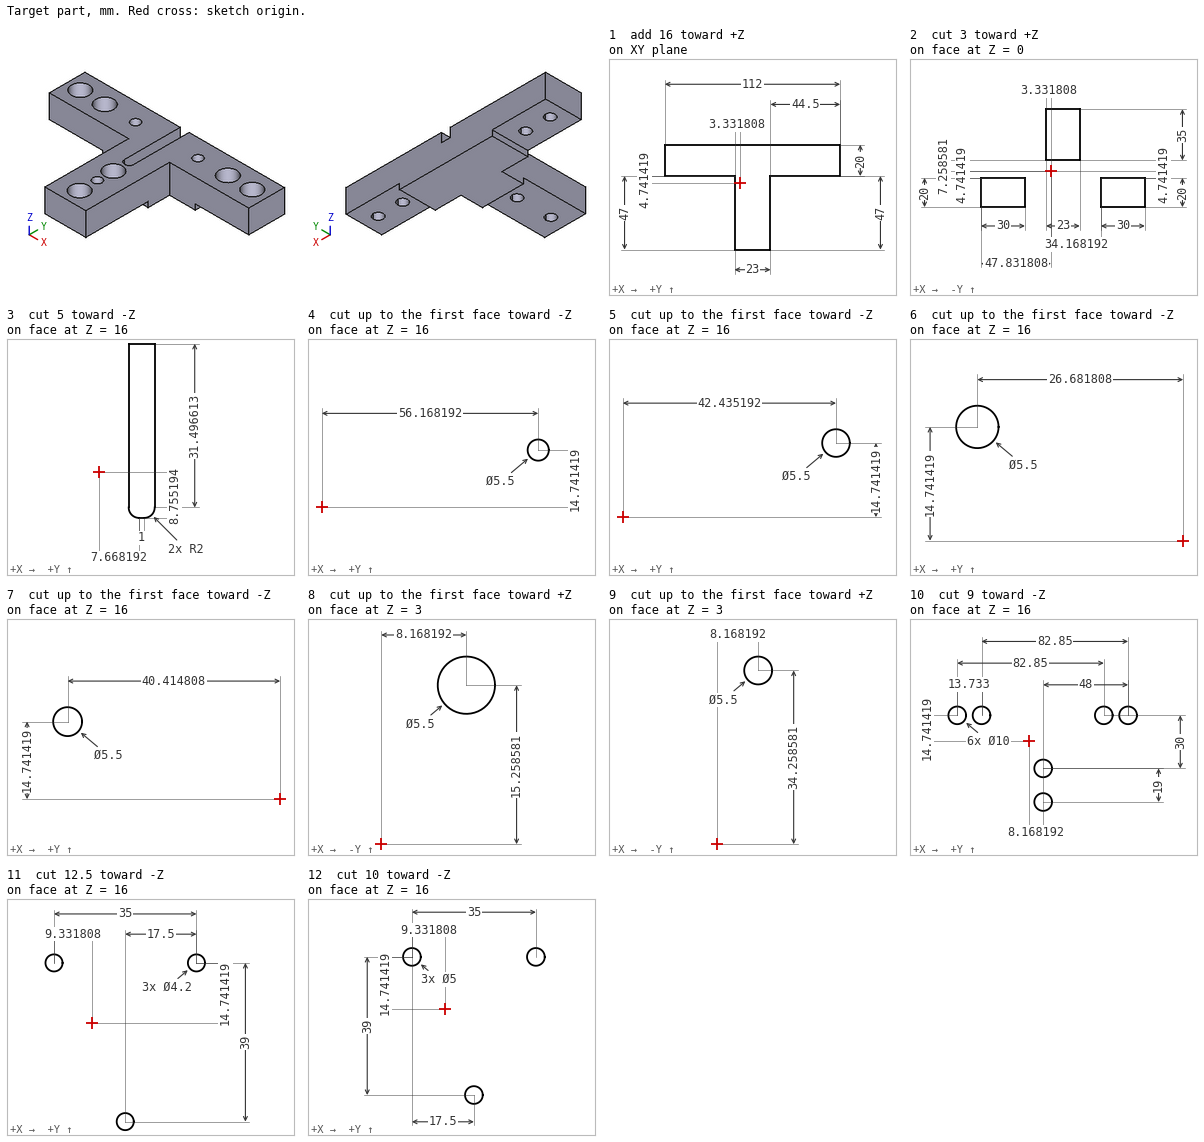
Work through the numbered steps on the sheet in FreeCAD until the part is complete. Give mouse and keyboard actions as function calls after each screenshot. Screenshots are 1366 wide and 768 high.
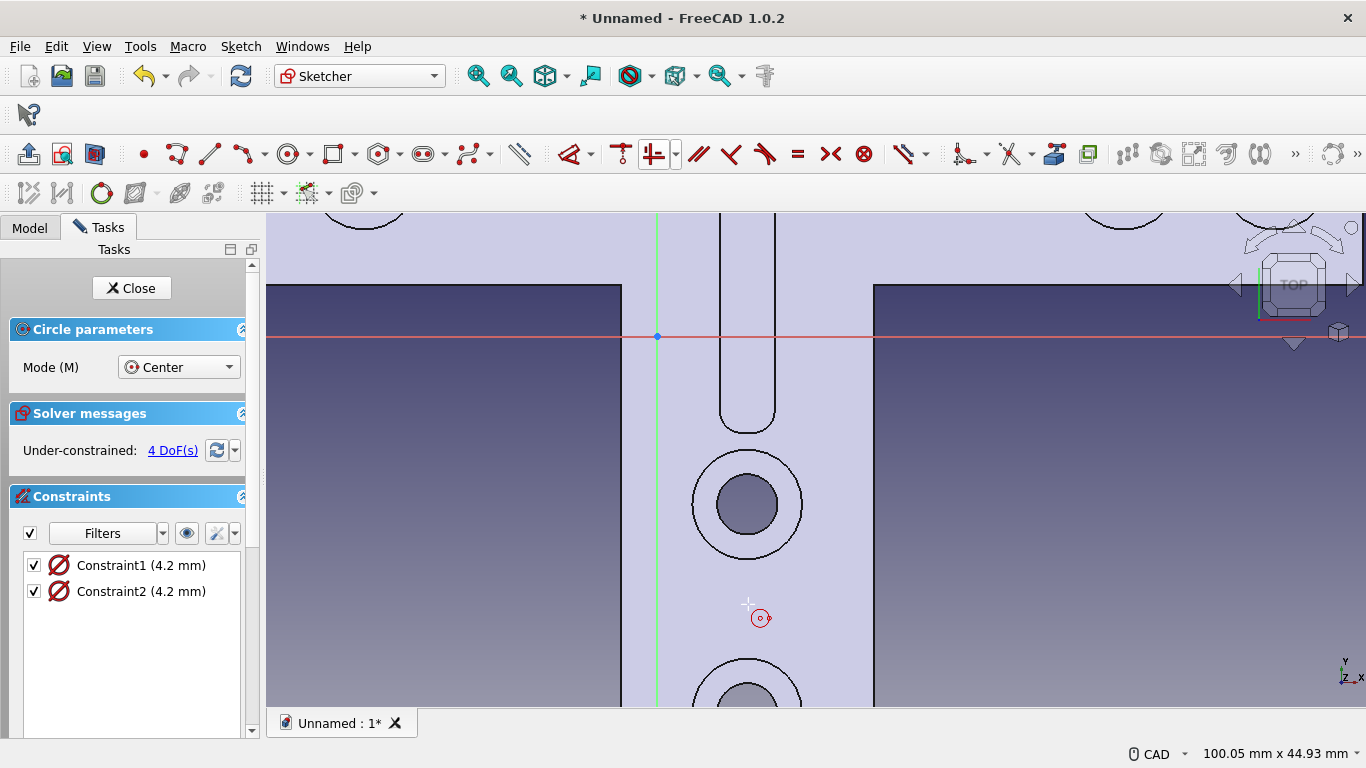
click(747, 603)
move(764, 587)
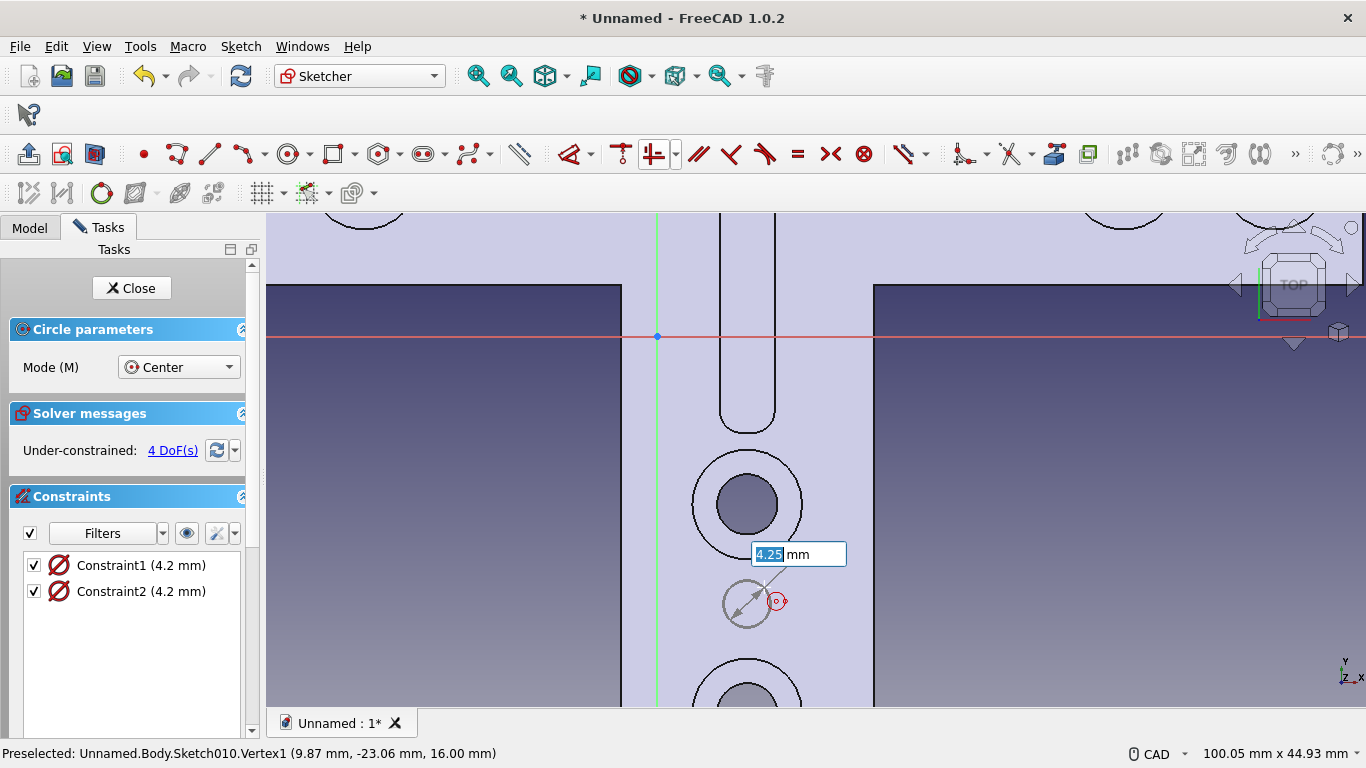
text(4.2)
key(Return)
key(Escape)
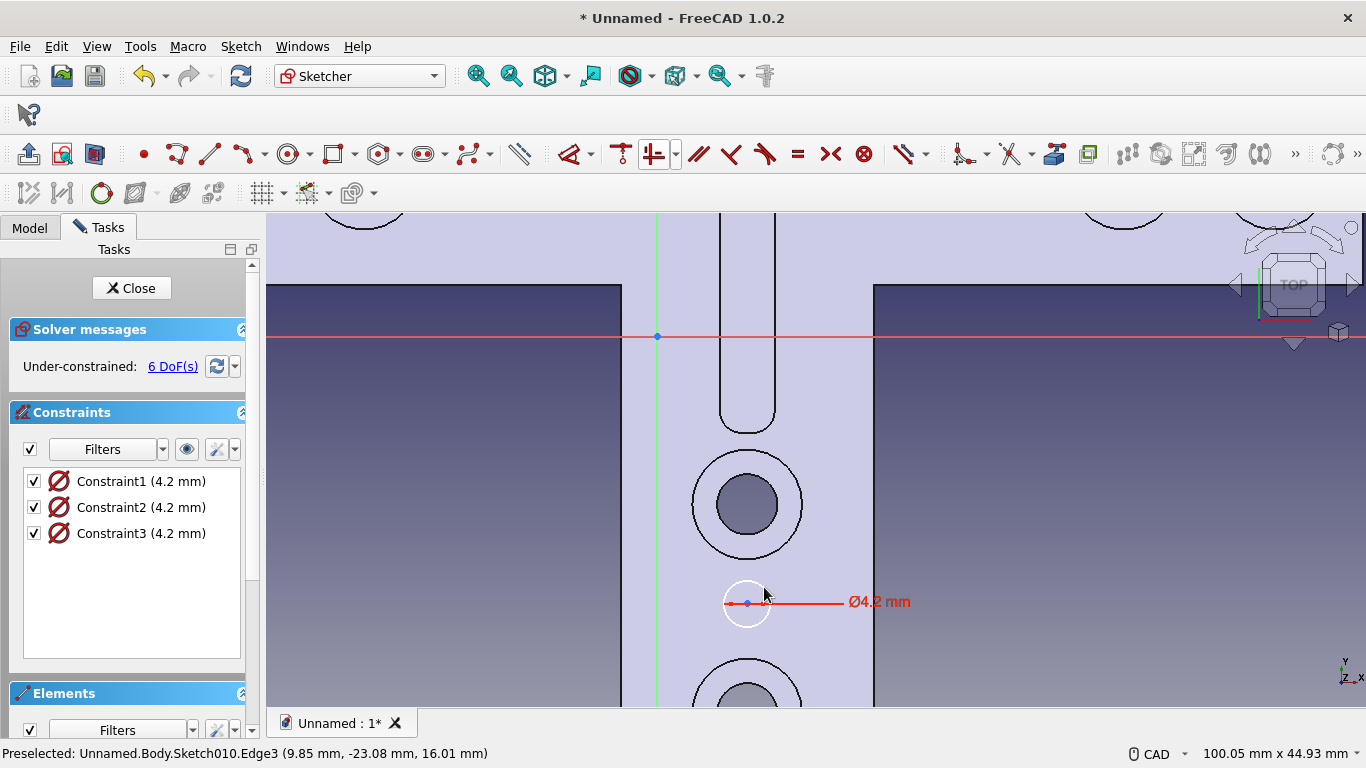
scroll(748, 604, down, 2)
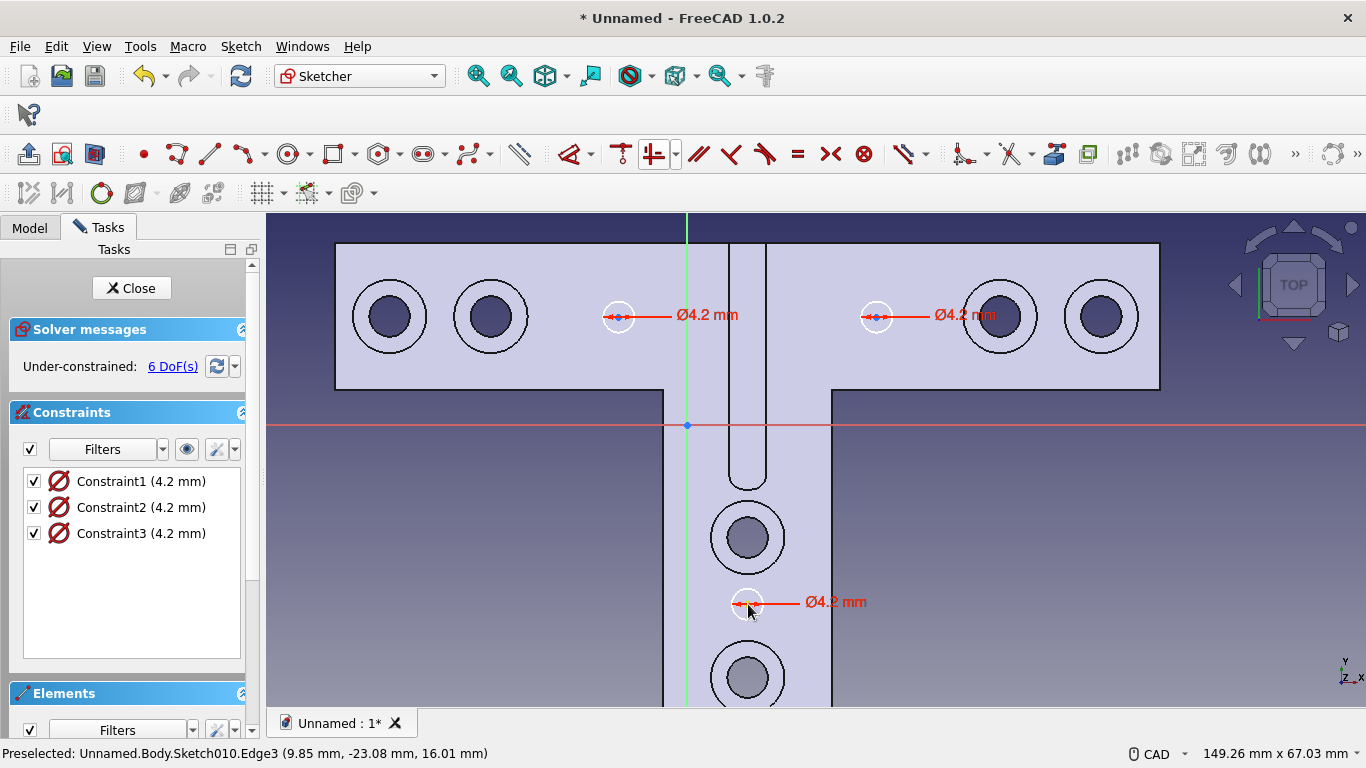
click(877, 317)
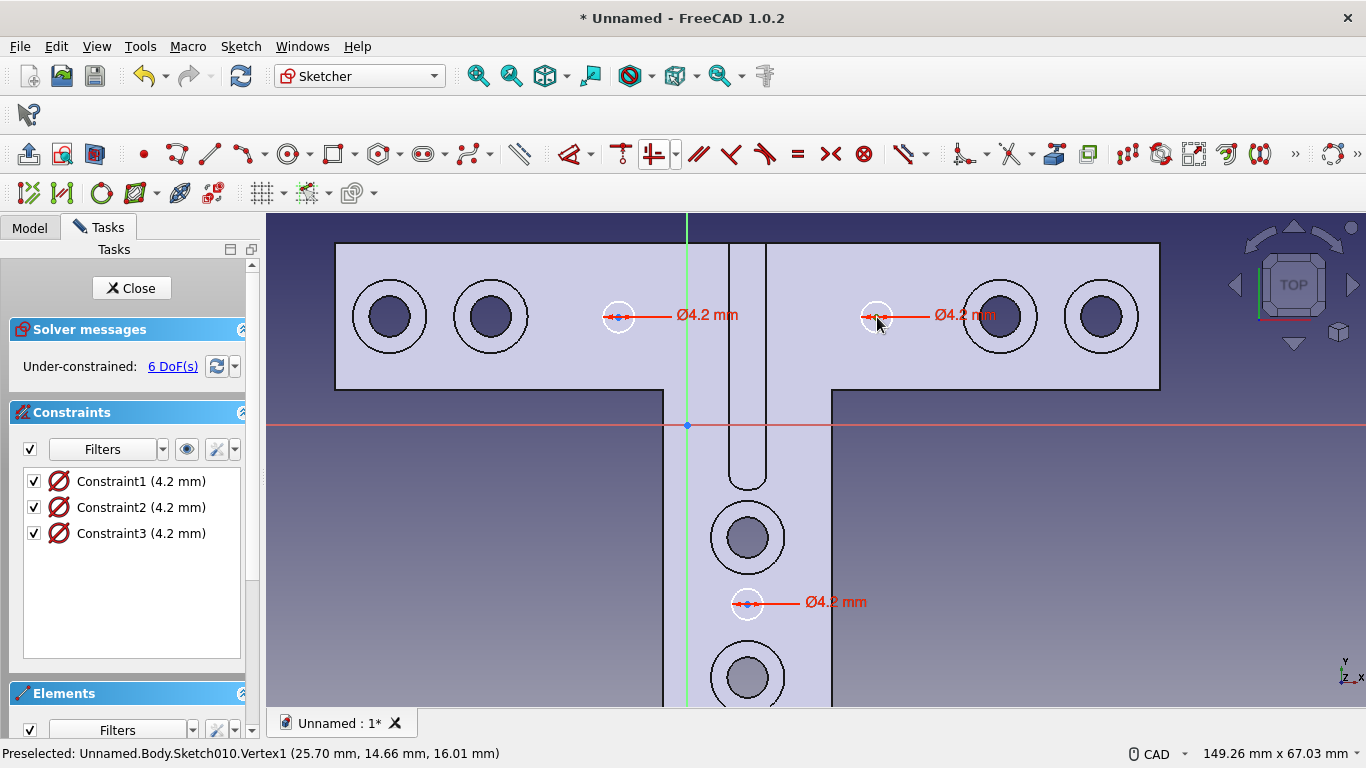
click(619, 317)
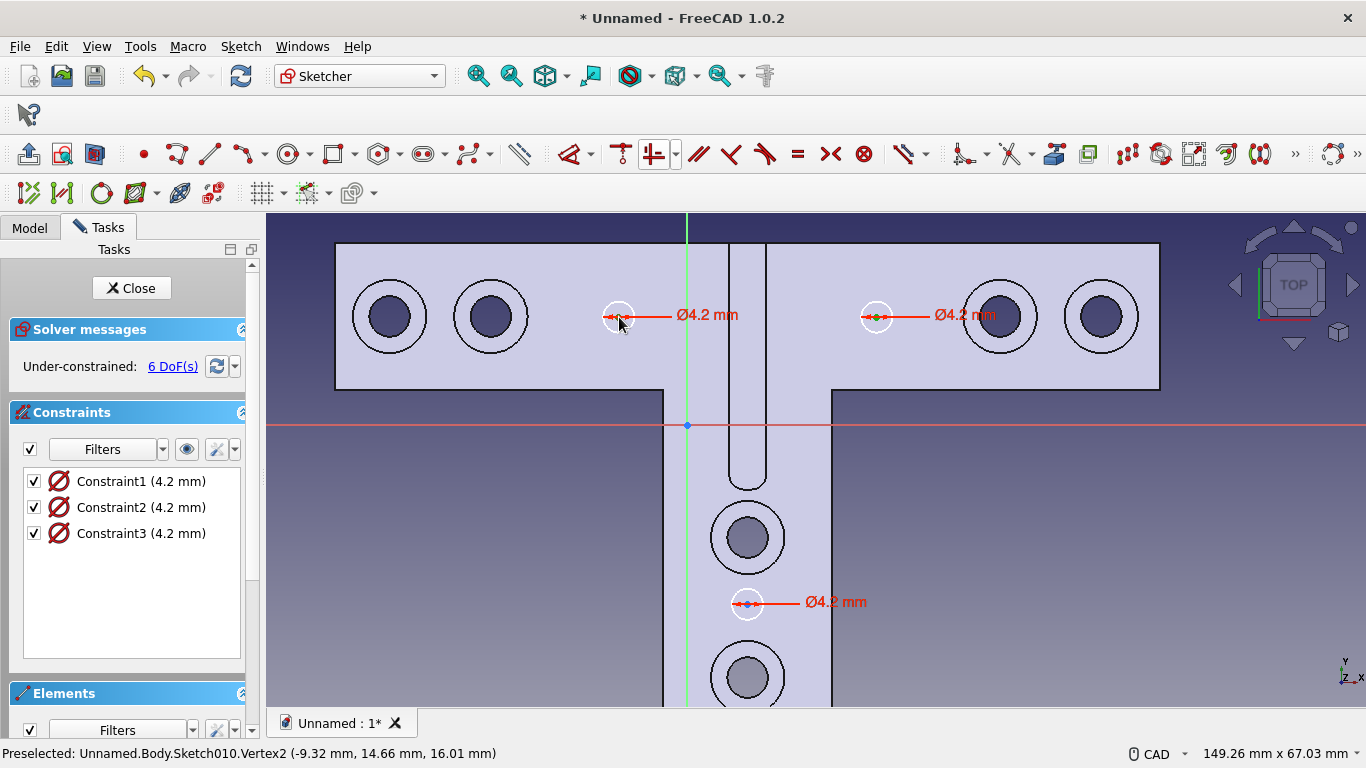
click(676, 154)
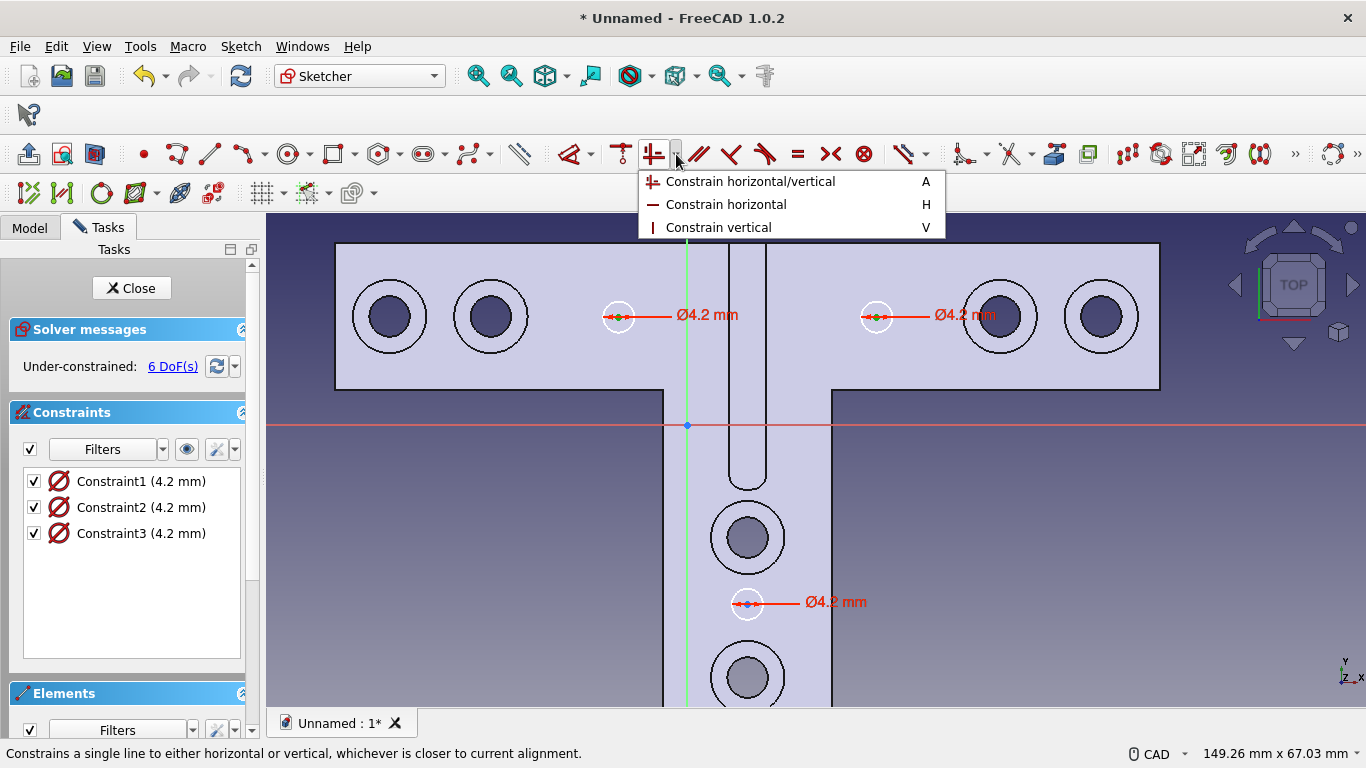
click(792, 204)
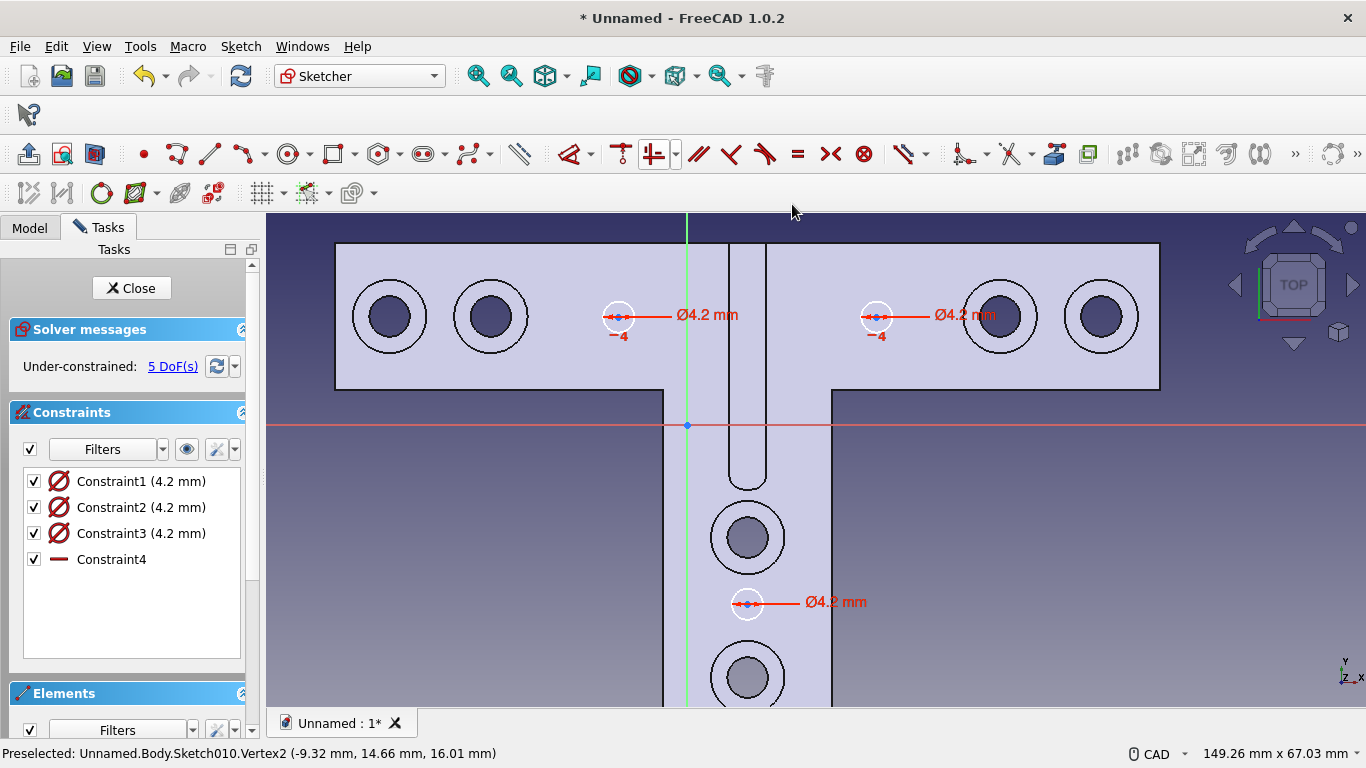
click(568, 154)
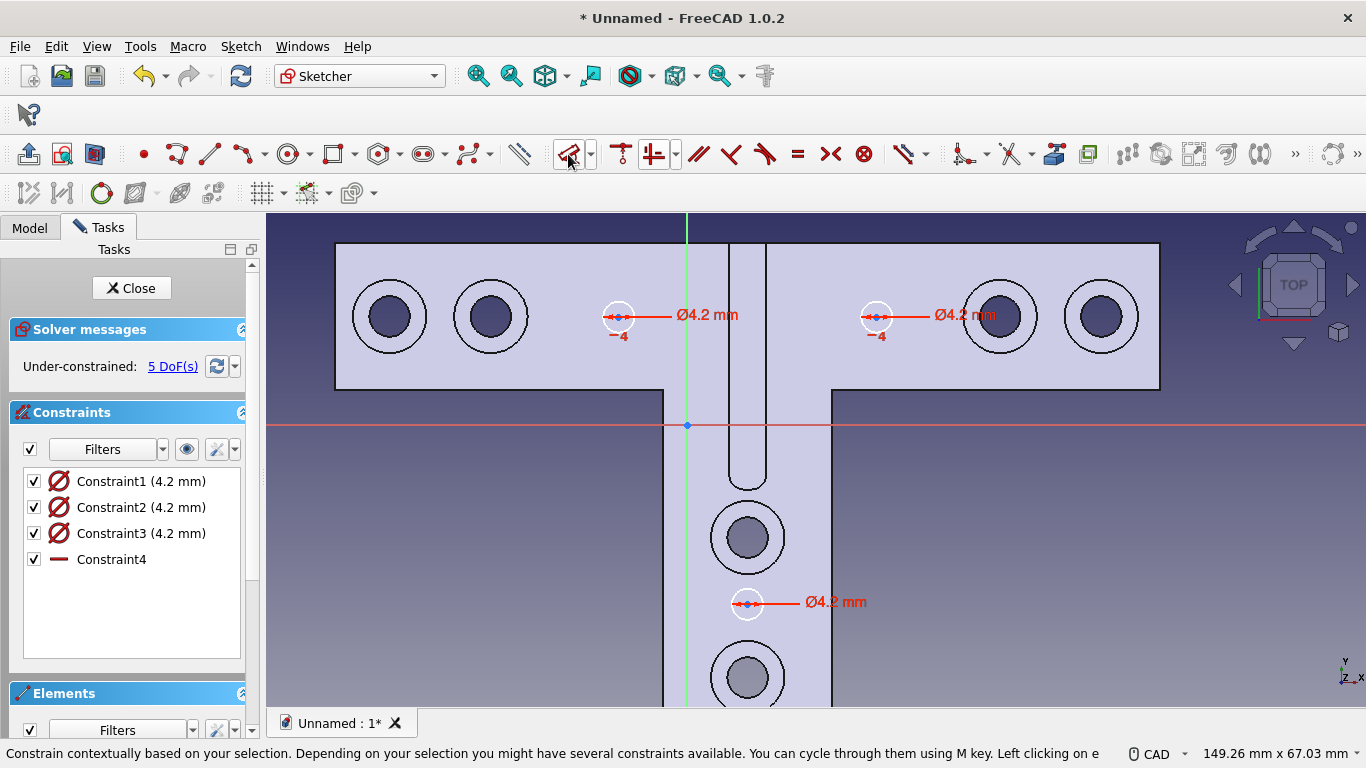
click(877, 317)